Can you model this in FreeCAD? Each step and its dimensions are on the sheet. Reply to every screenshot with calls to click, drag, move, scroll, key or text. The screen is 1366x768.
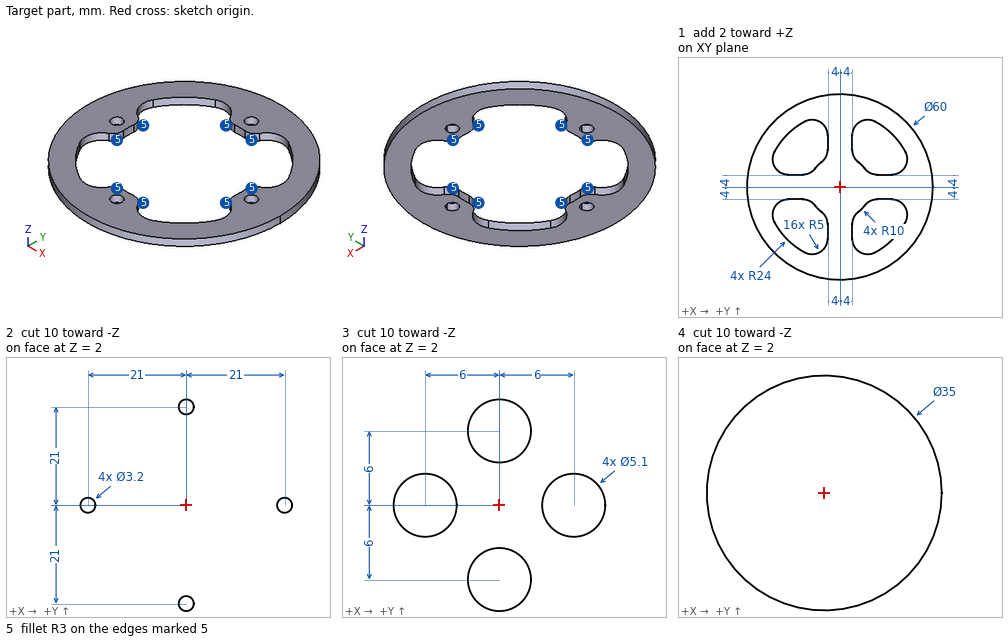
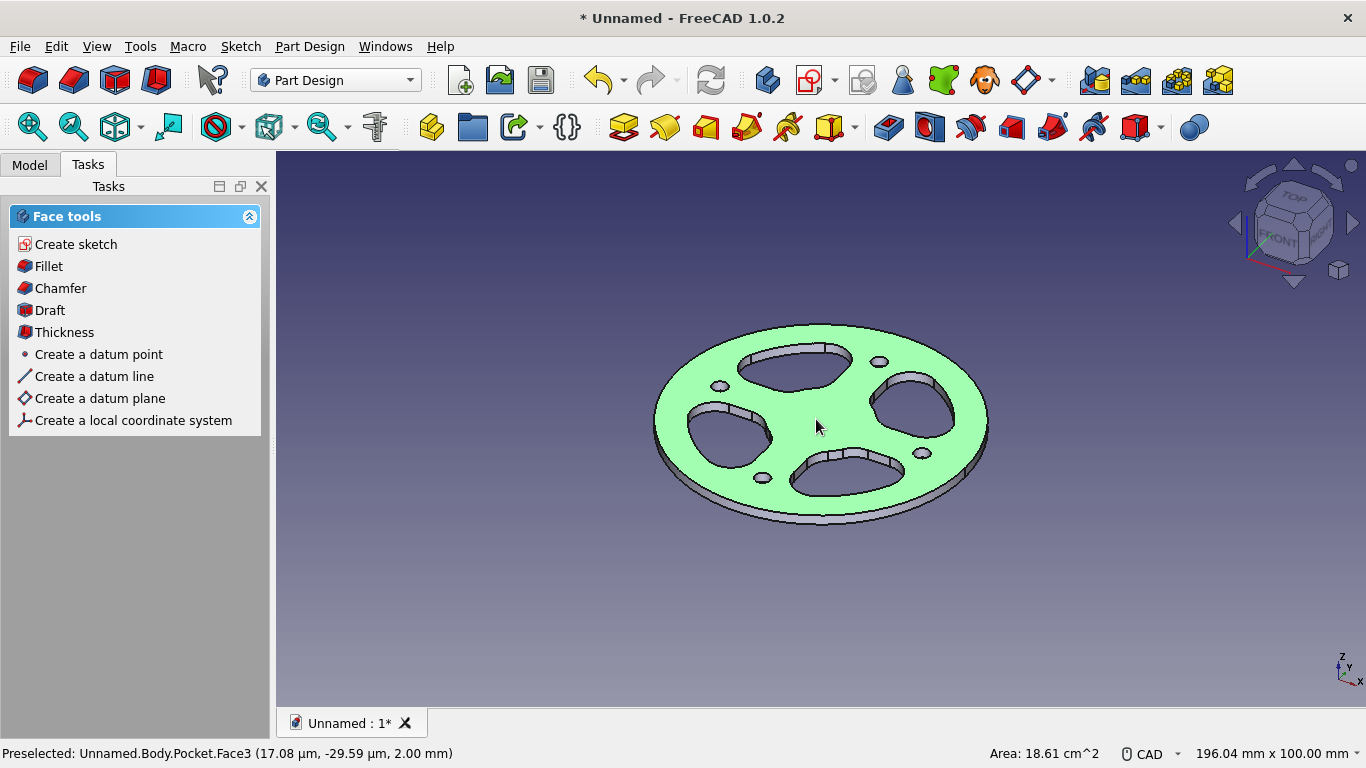
click(808, 80)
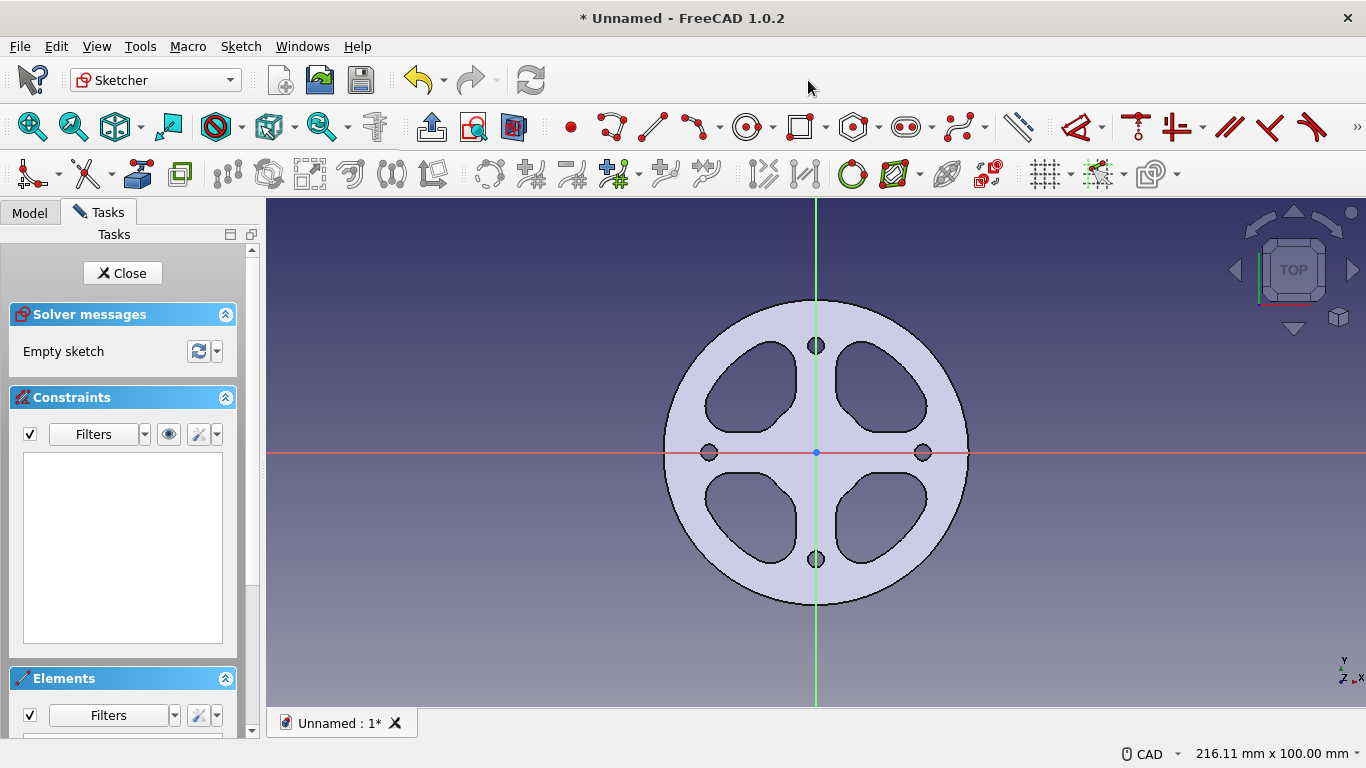
scroll(838, 452, up, 7)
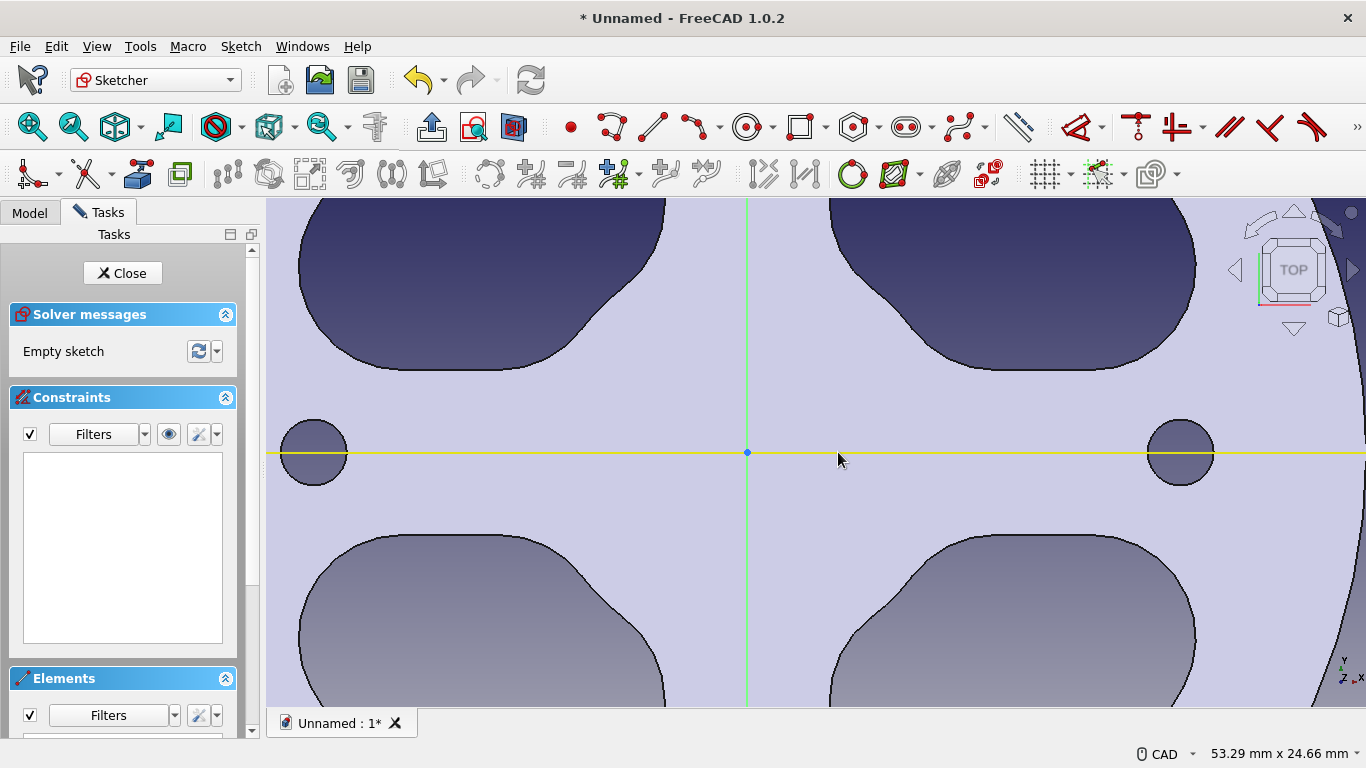
key(g)
key(c)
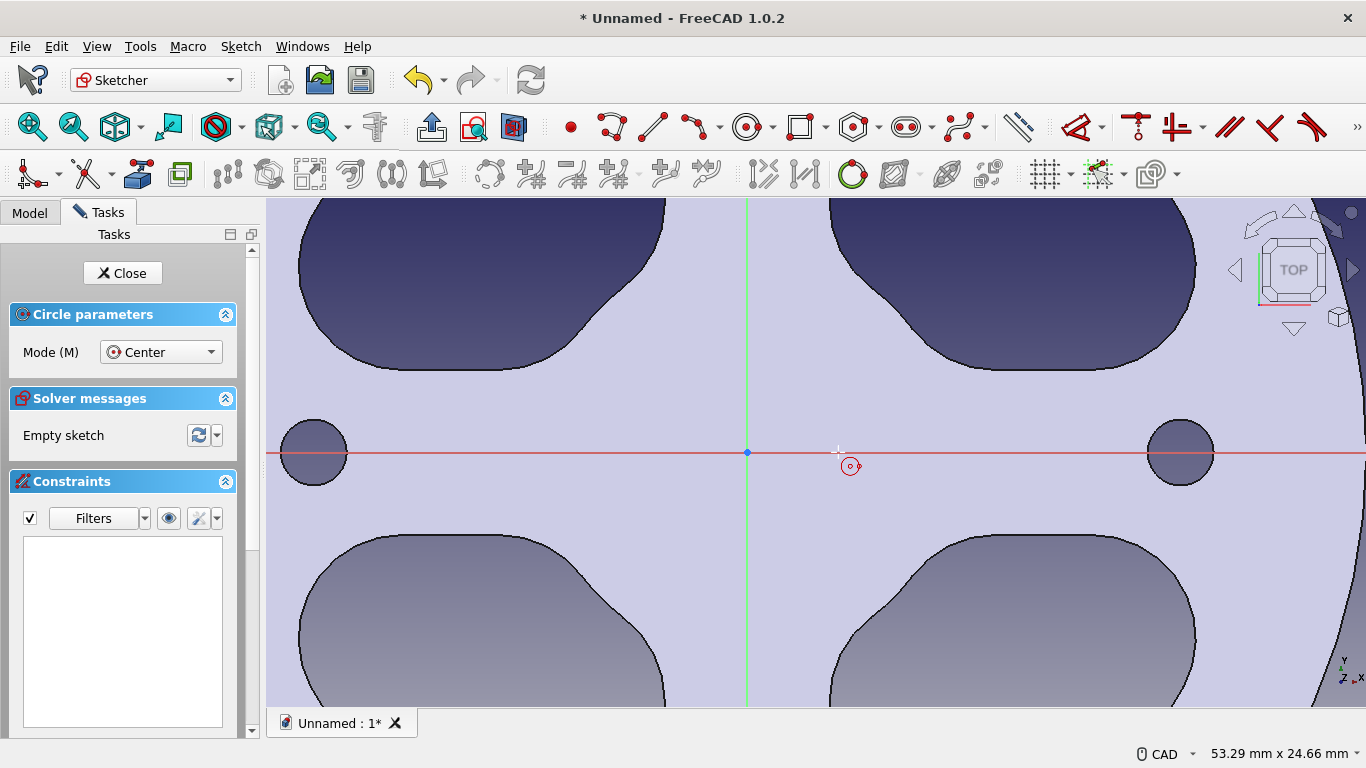
click(747, 329)
click(784, 291)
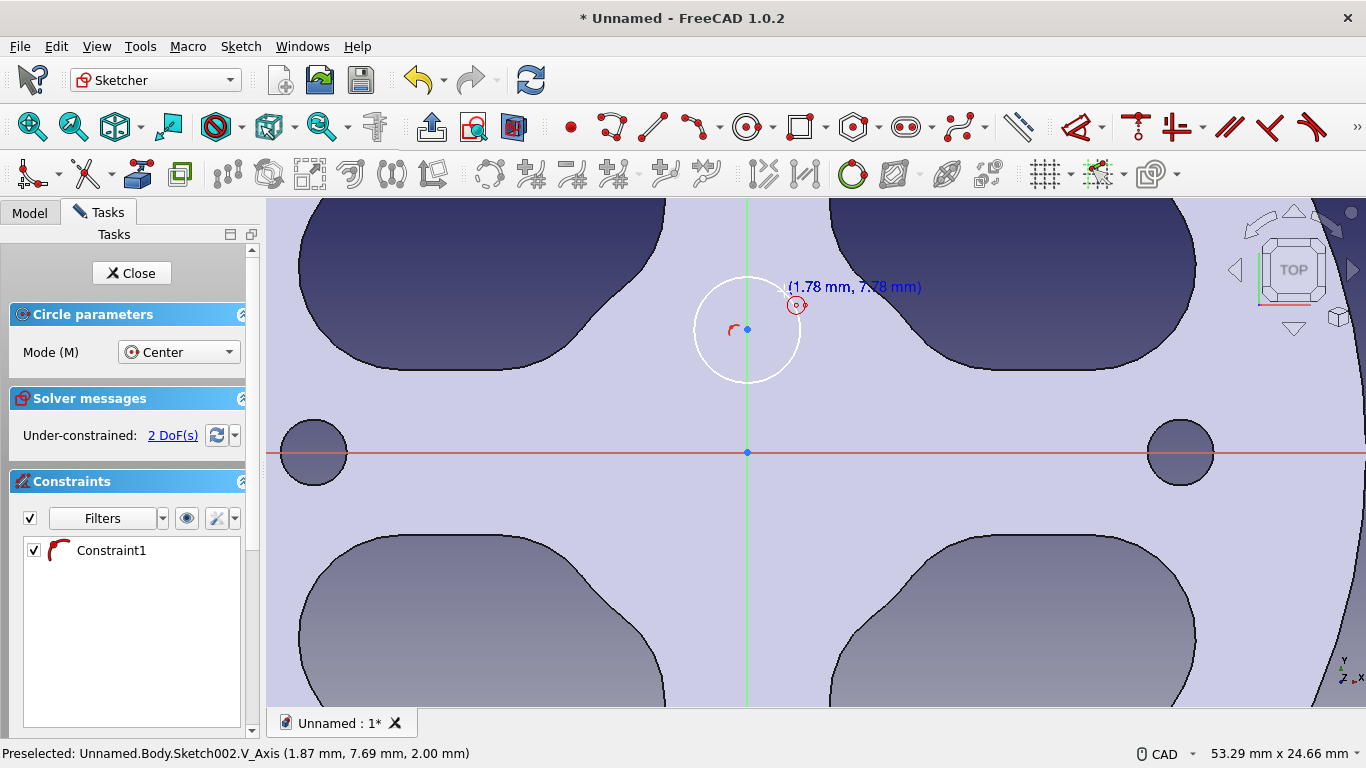
click(623, 452)
click(661, 415)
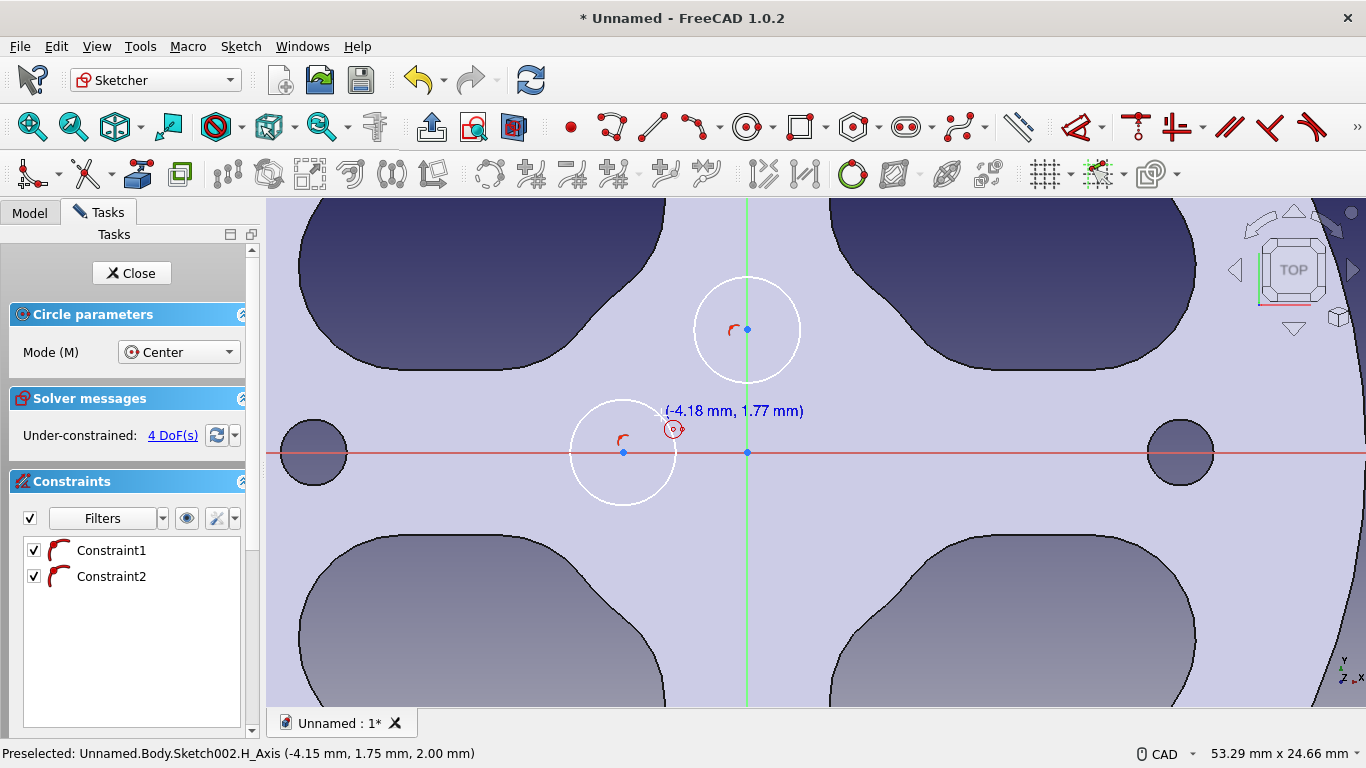
click(871, 452)
click(908, 415)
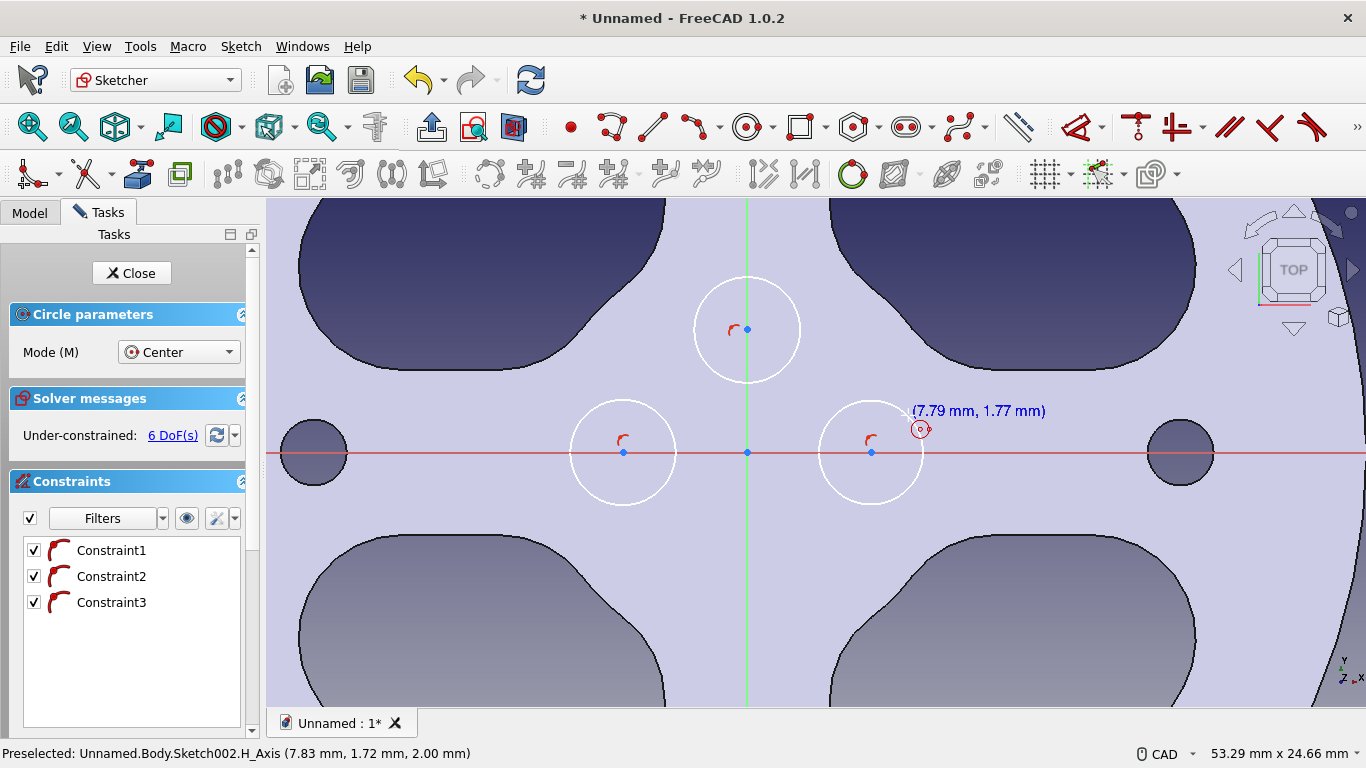
click(747, 576)
click(784, 539)
key(Escape)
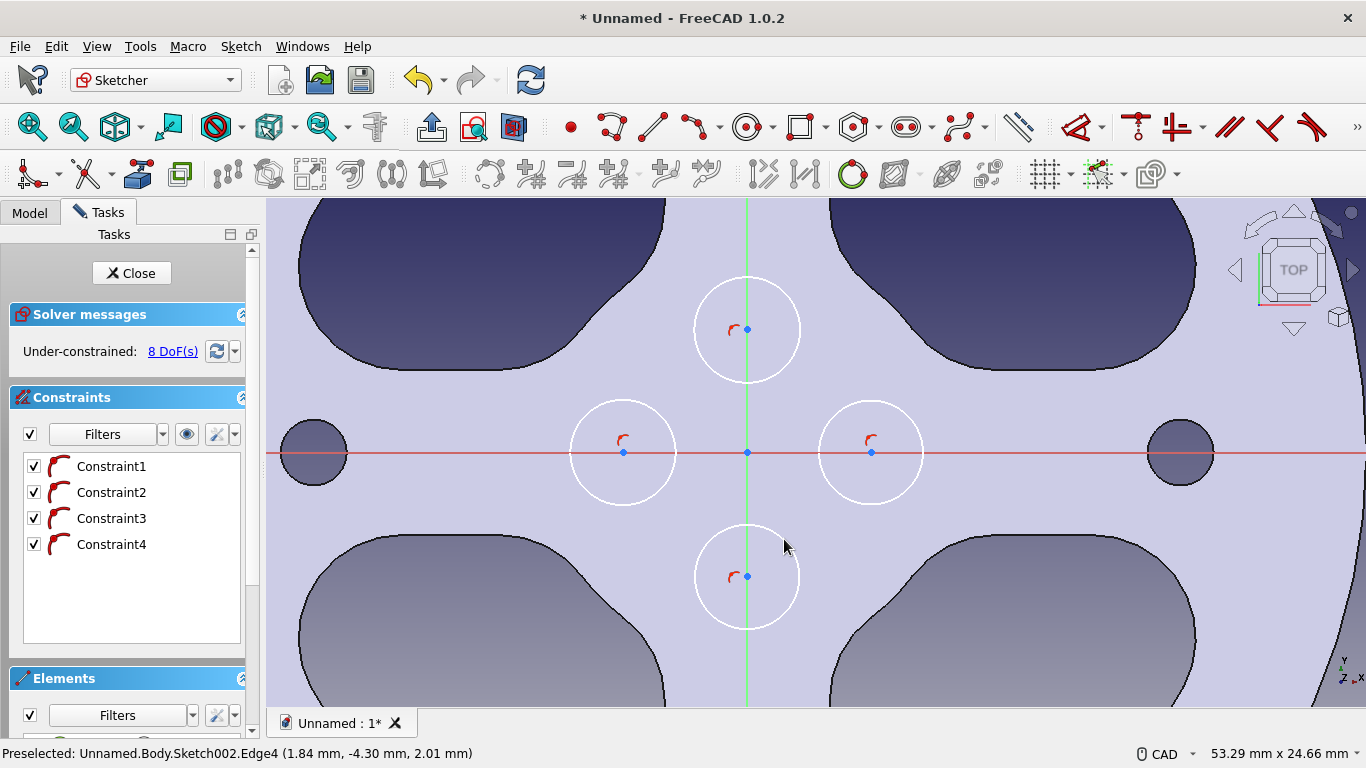
click(784, 292)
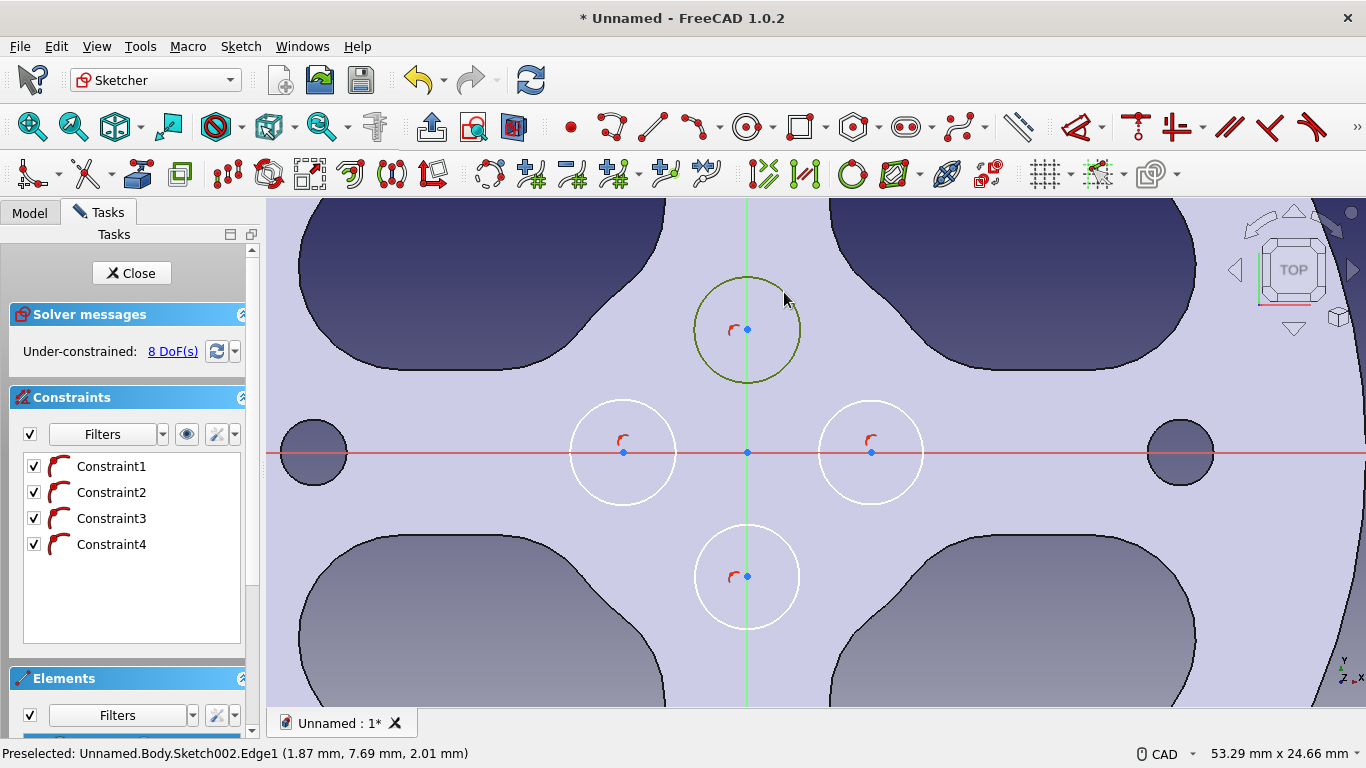
click(660, 415)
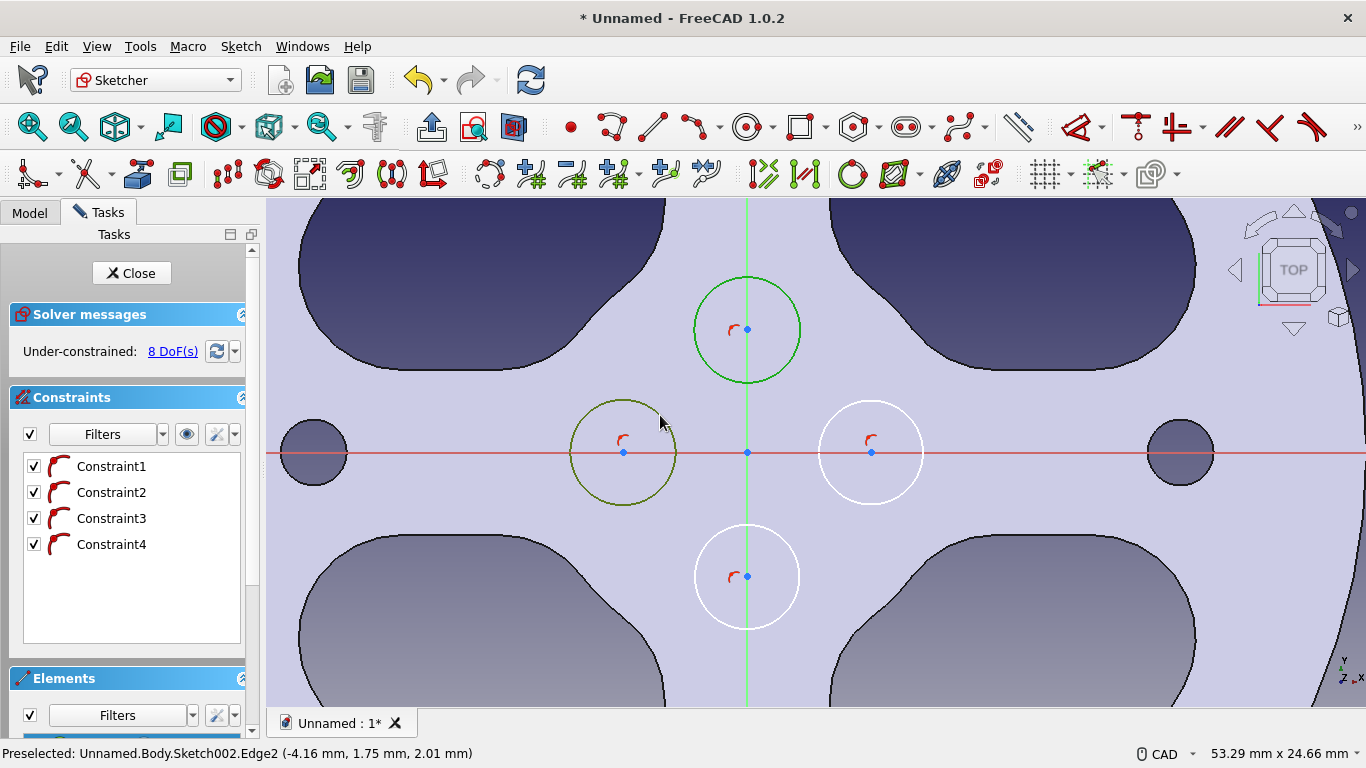
click(908, 416)